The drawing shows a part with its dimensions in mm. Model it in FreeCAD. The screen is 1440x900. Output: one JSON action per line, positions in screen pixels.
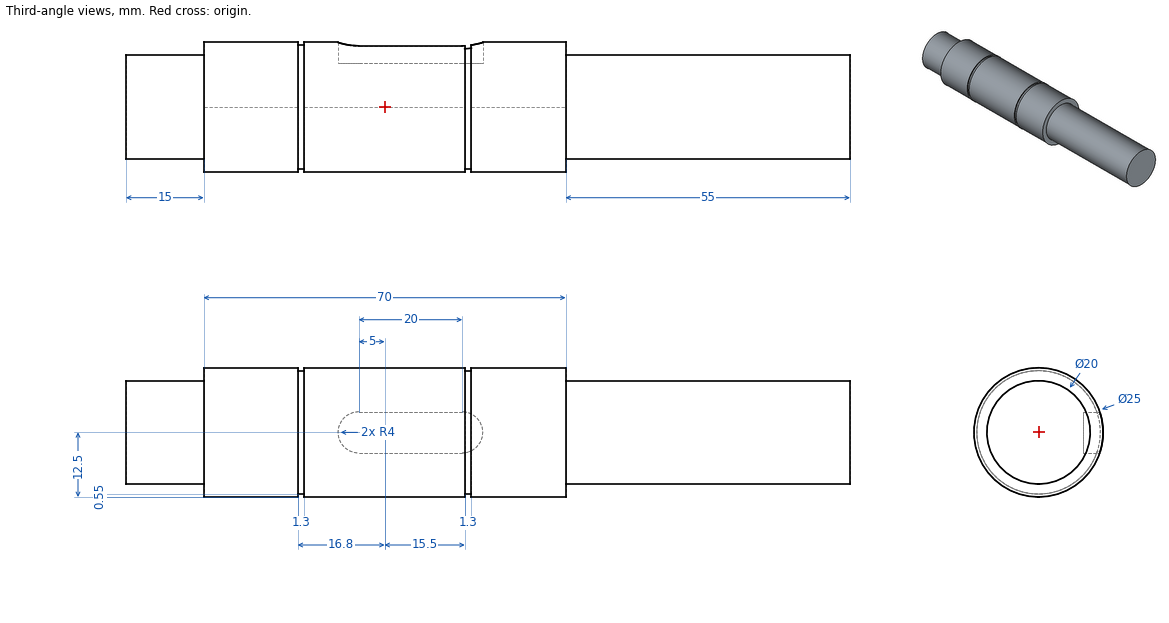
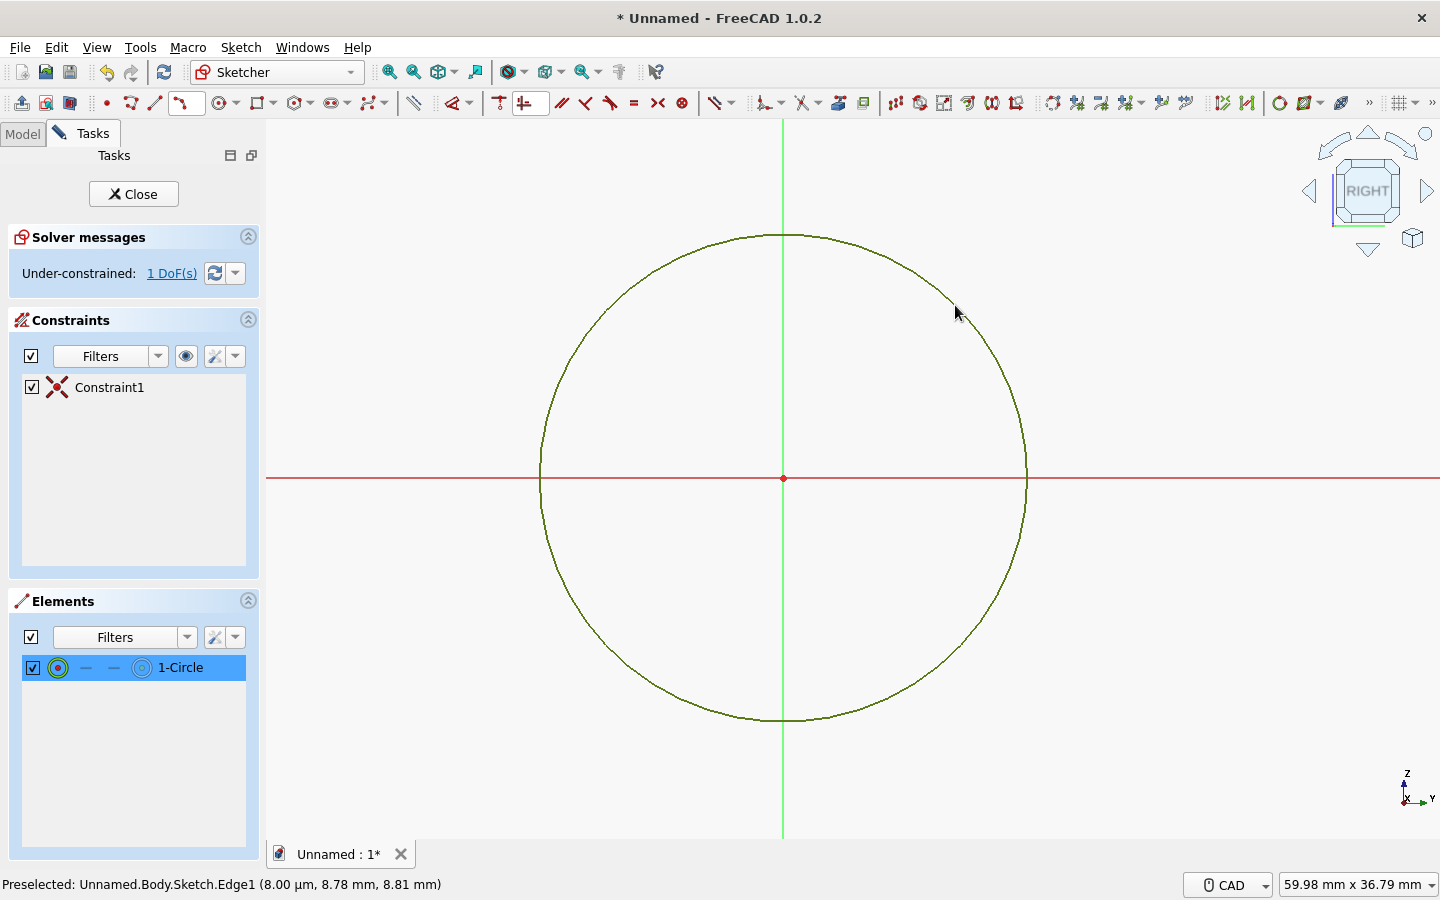
{"action": "left_click", "coordinate": [472, 104]}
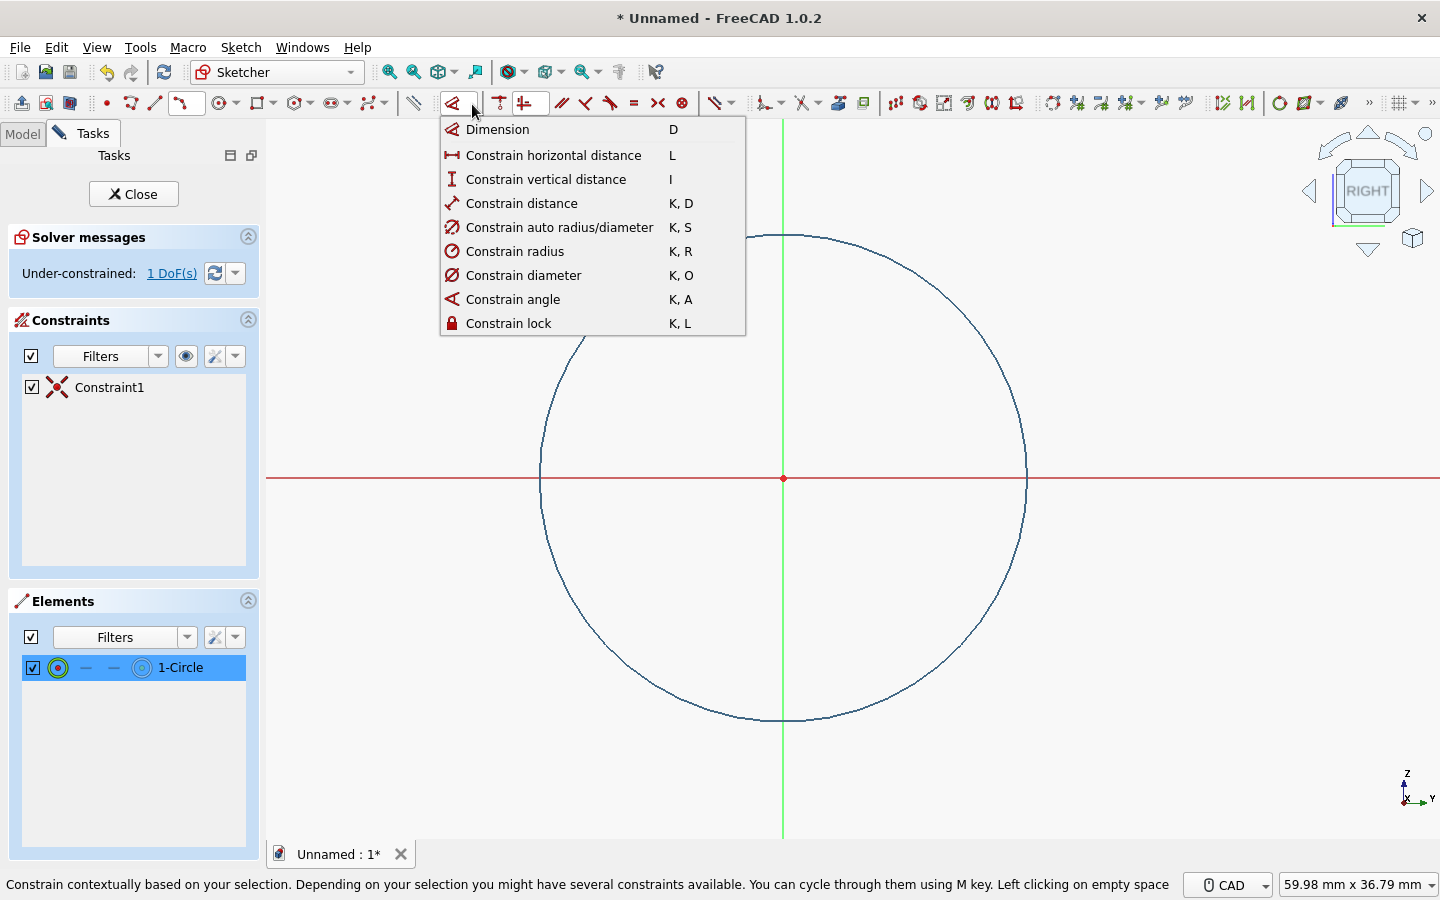
{"action": "left_click", "coordinate": [593, 275]}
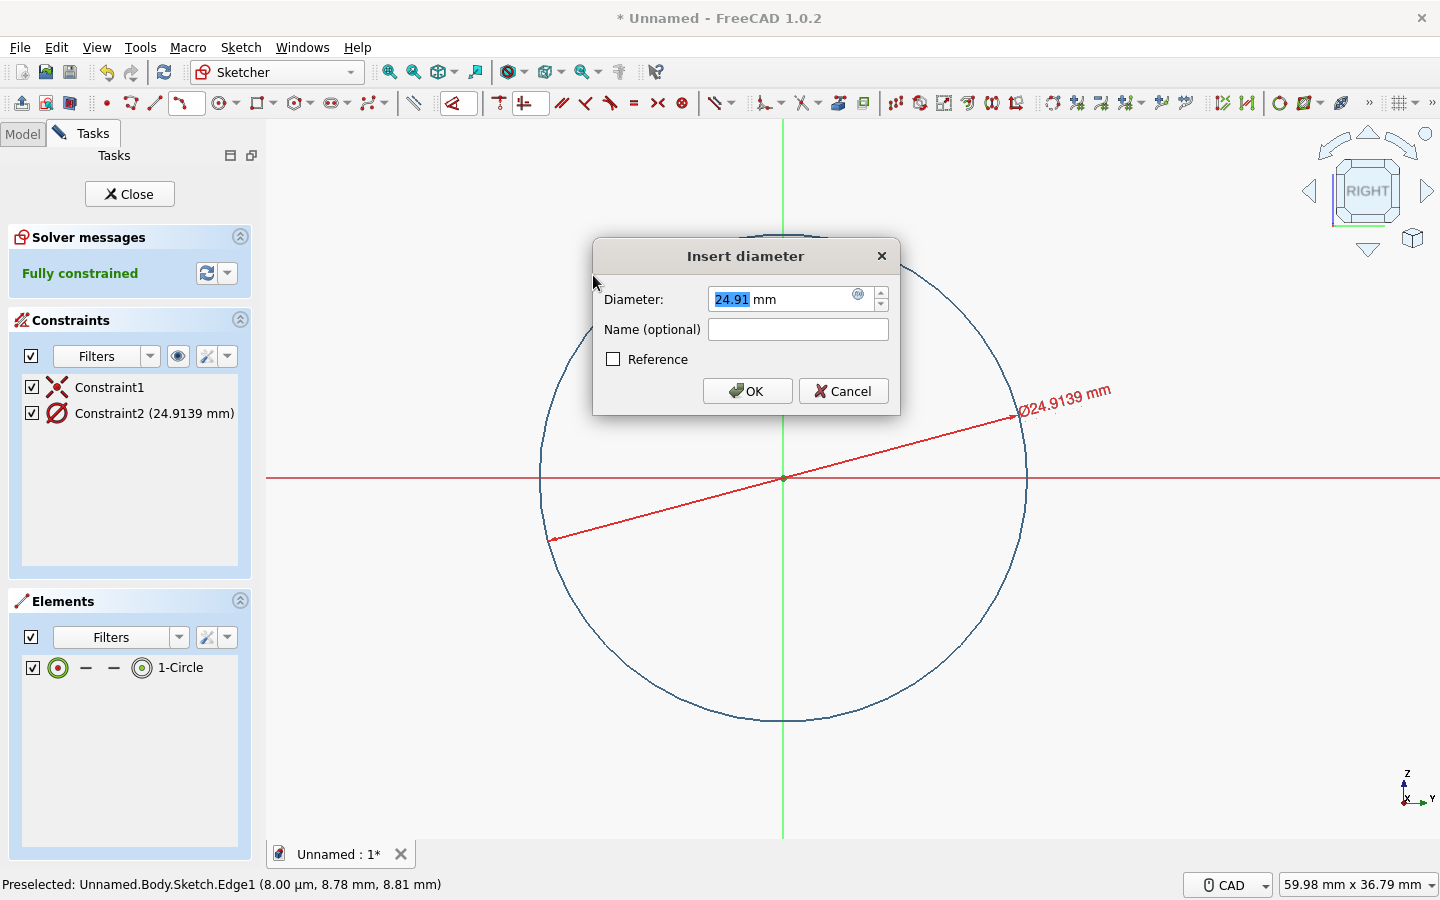
{"action": "type", "text": "25"}
{"action": "key", "text": "Return"}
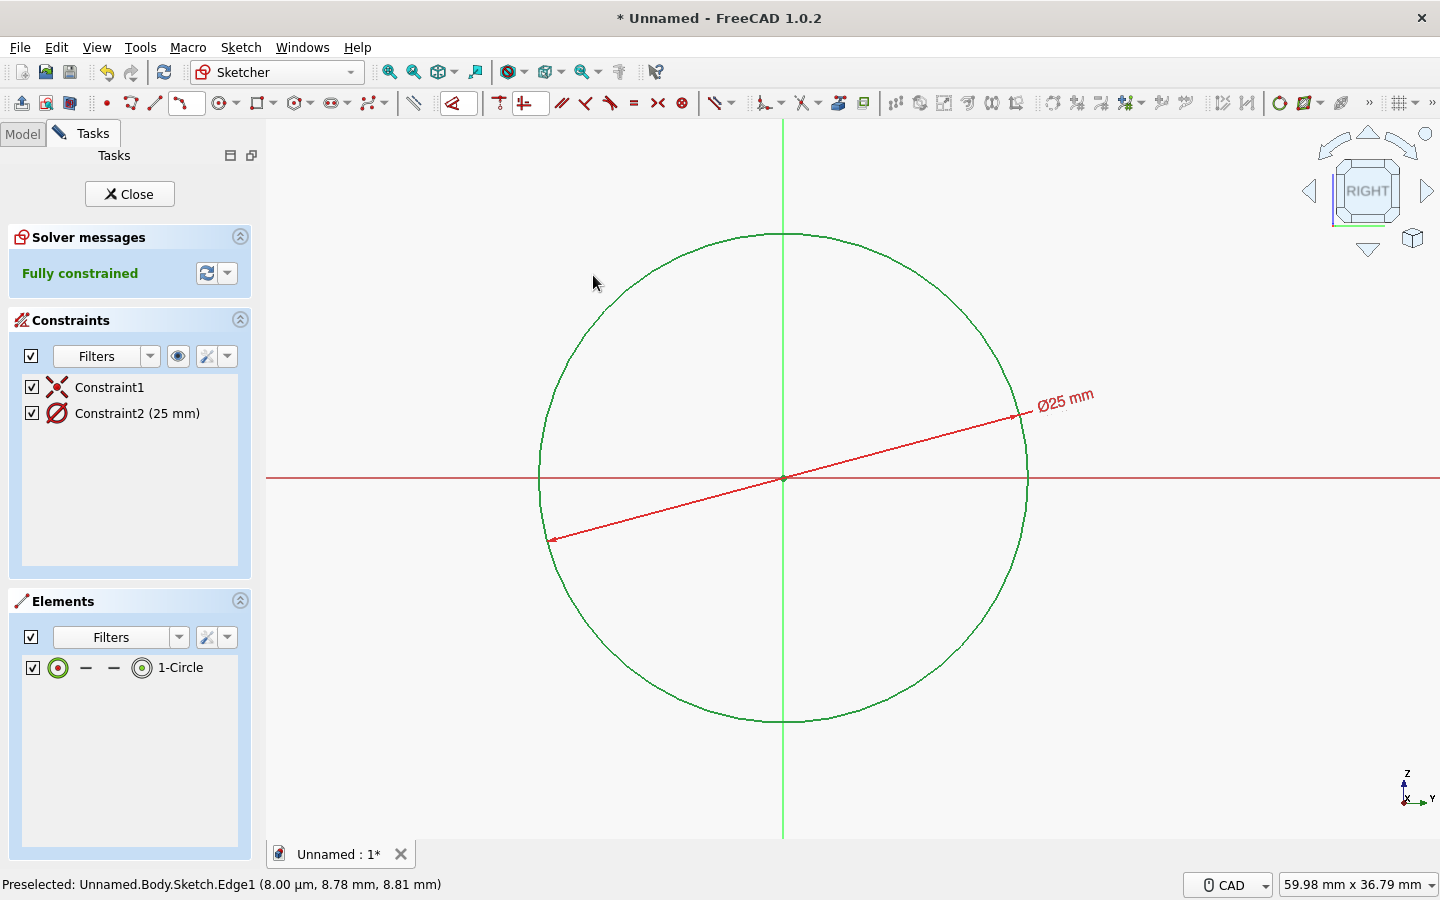
{"action": "left_click", "coordinate": [130, 194]}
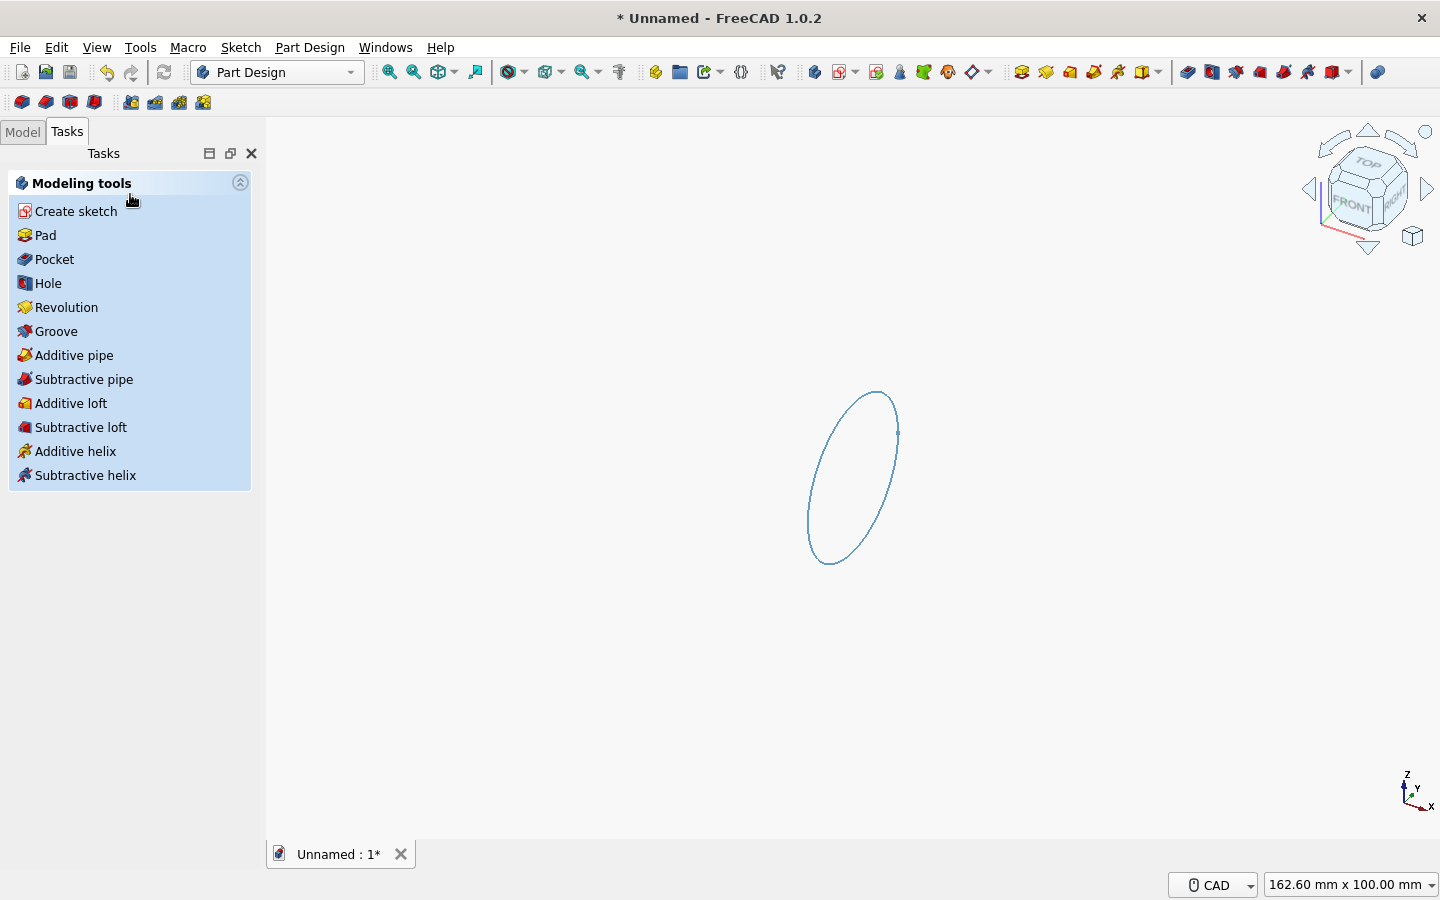
{"action": "left_click", "coordinate": [1022, 72]}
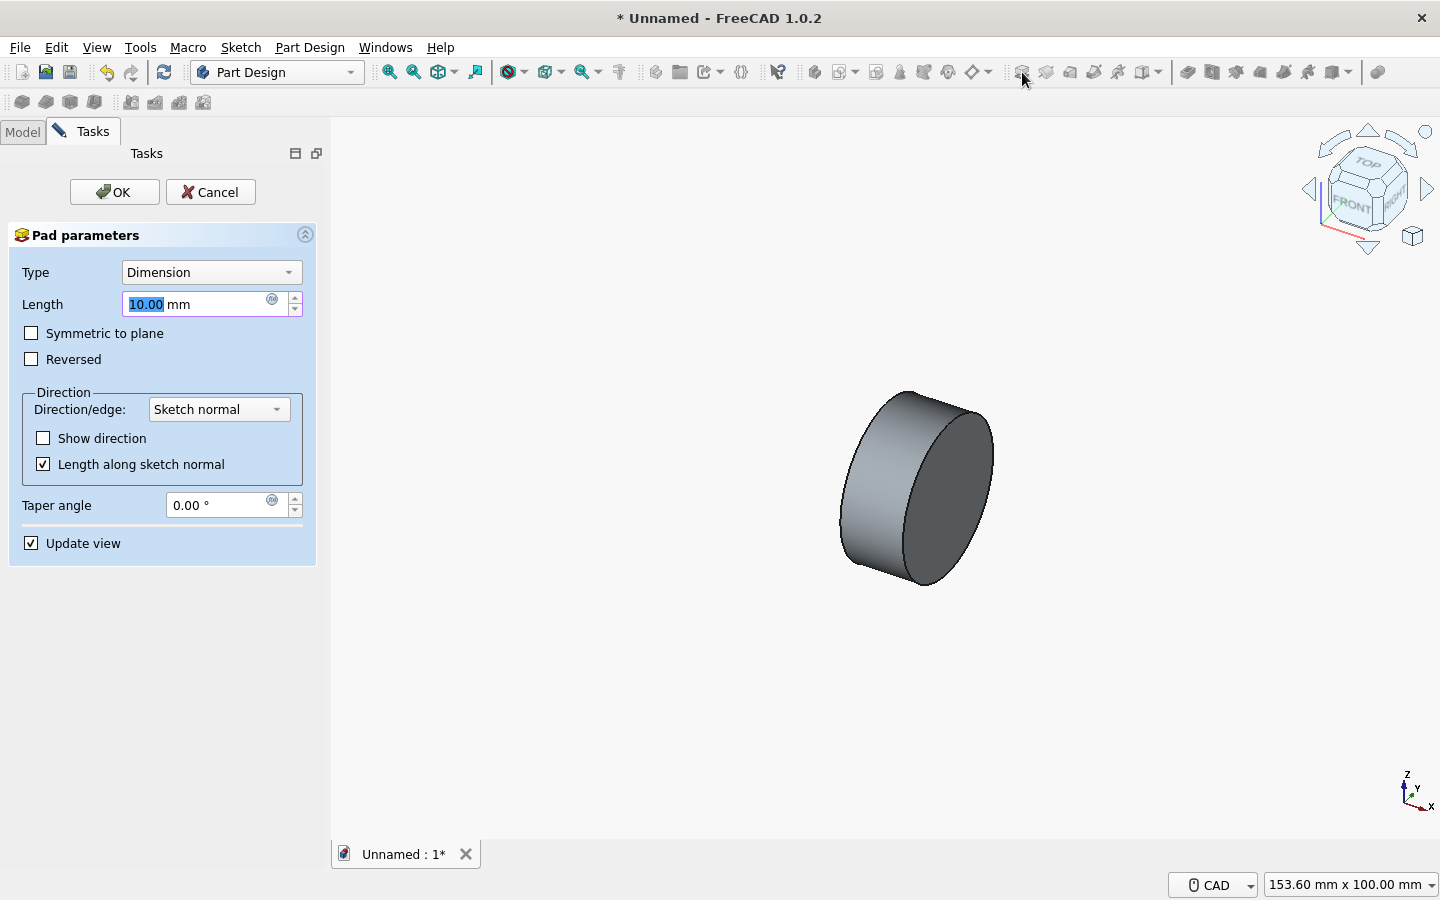
{"action": "type", "text": "70"}
{"action": "key", "text": "Tab"}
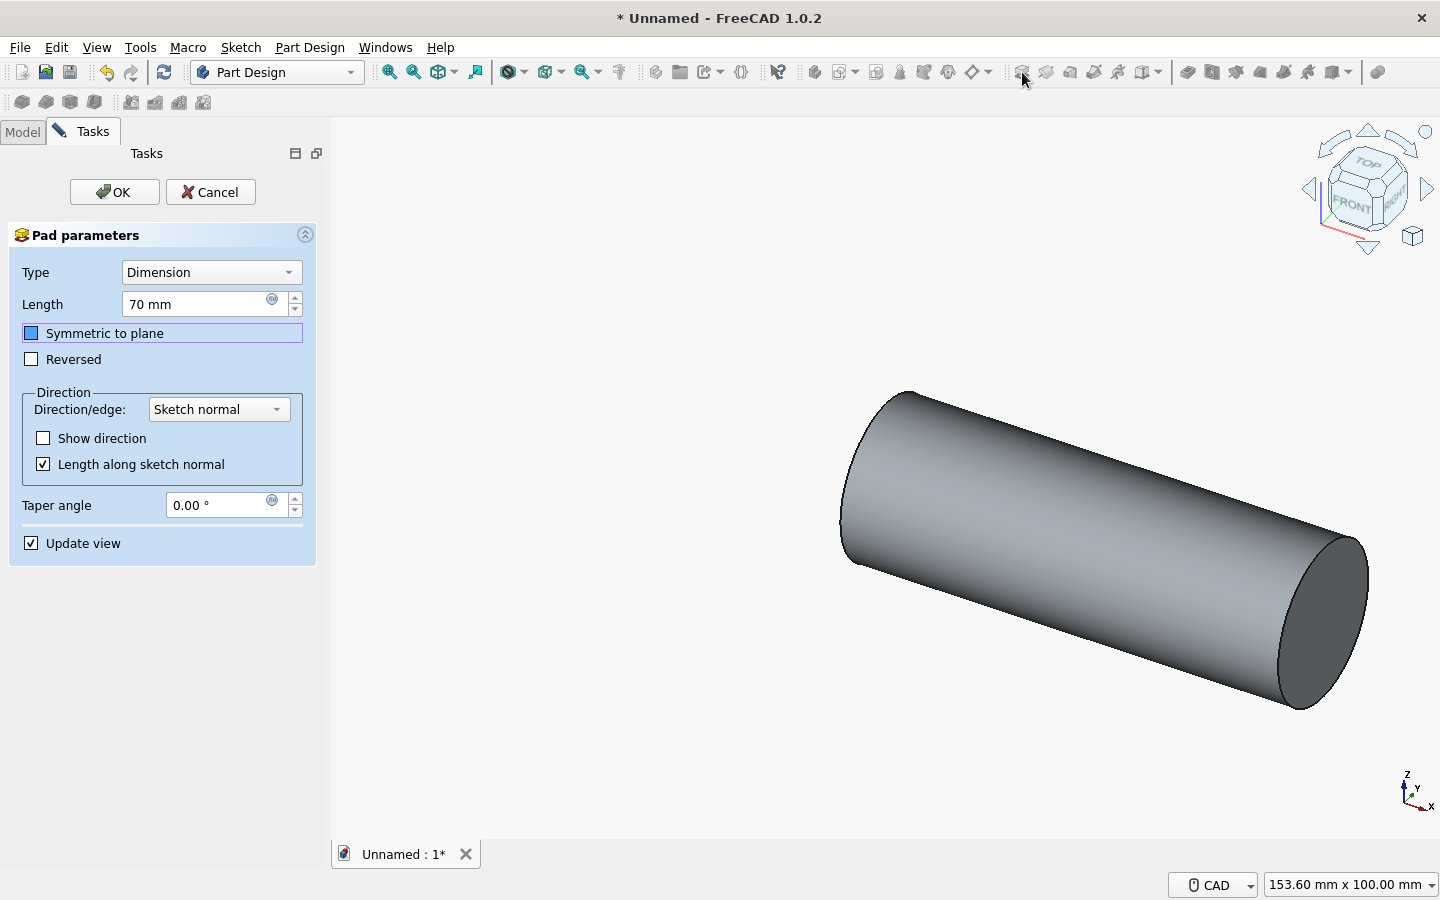
{"action": "left_click", "coordinate": [30, 333]}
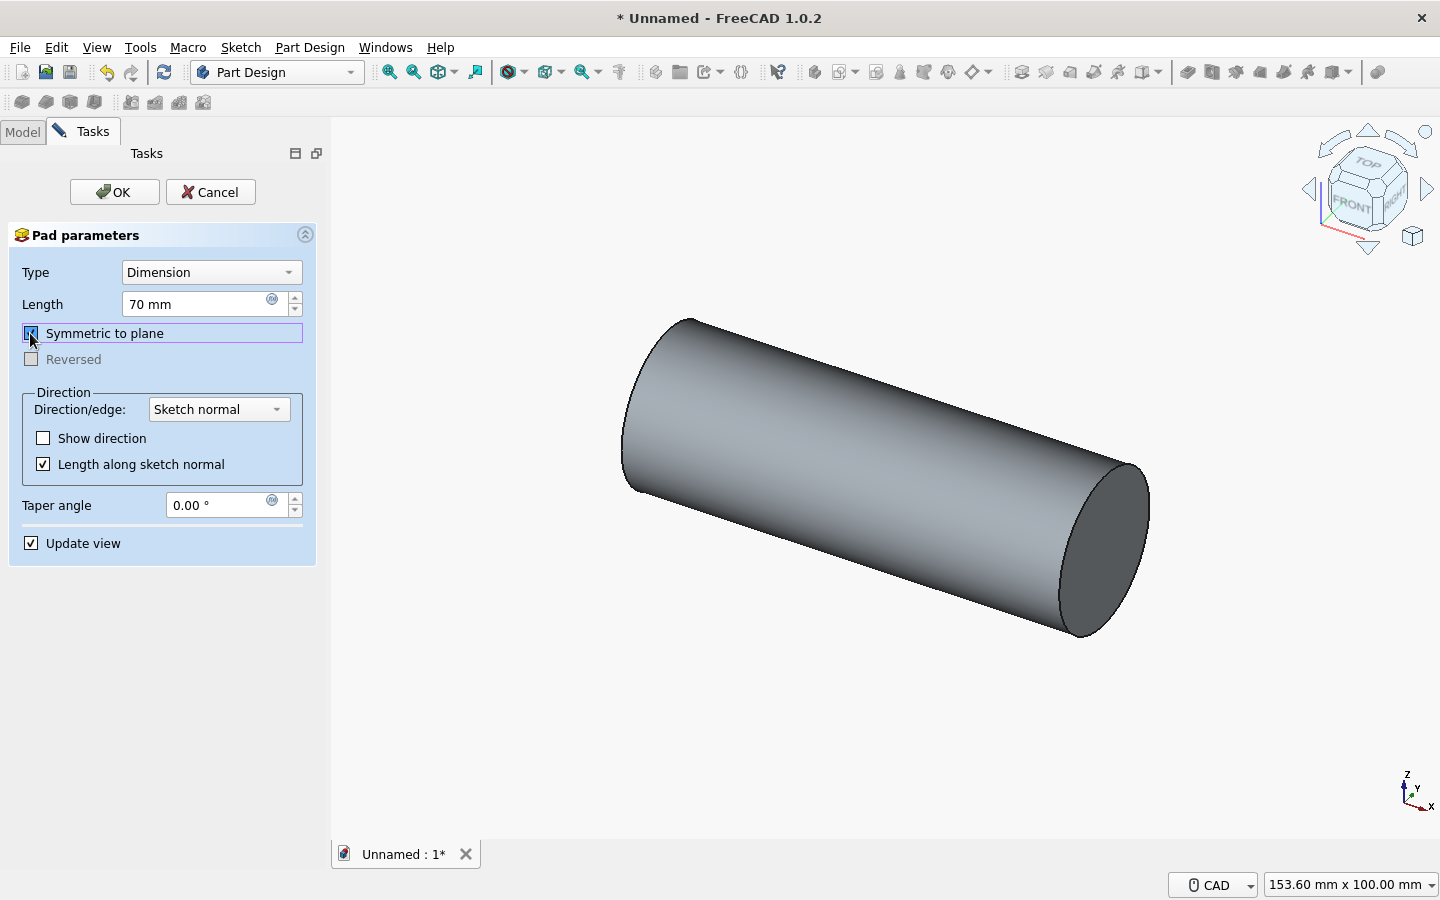
{"action": "left_click", "coordinate": [115, 192]}